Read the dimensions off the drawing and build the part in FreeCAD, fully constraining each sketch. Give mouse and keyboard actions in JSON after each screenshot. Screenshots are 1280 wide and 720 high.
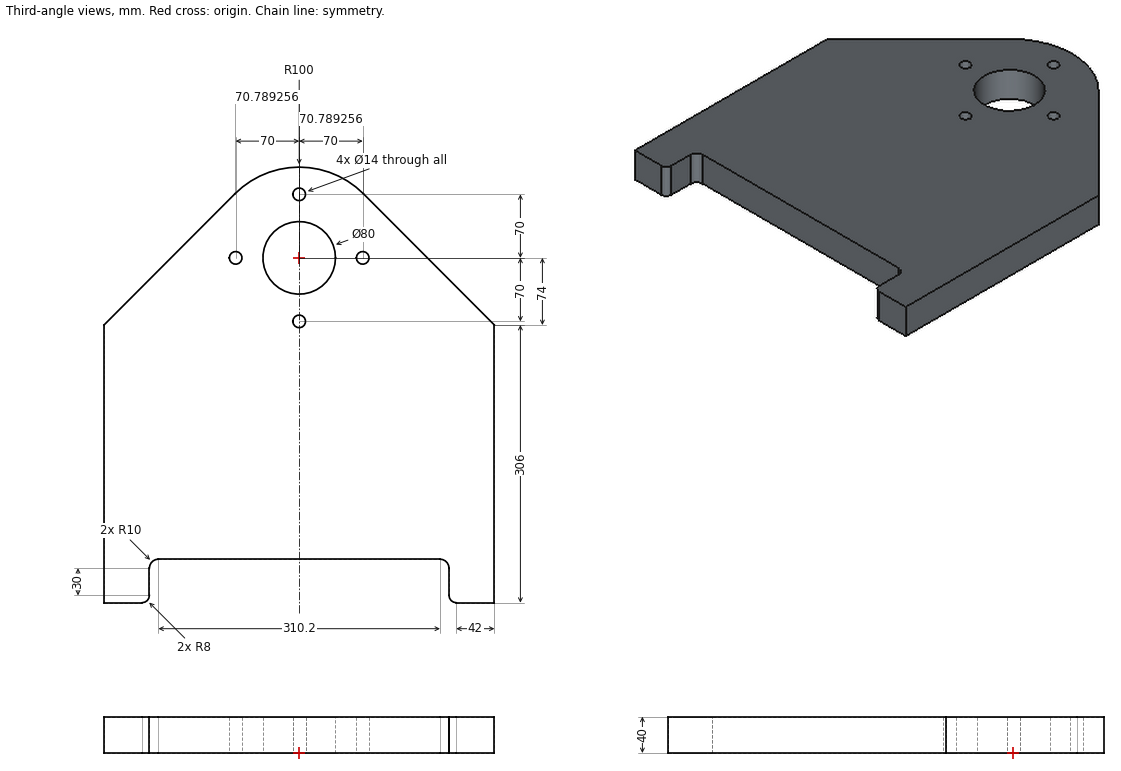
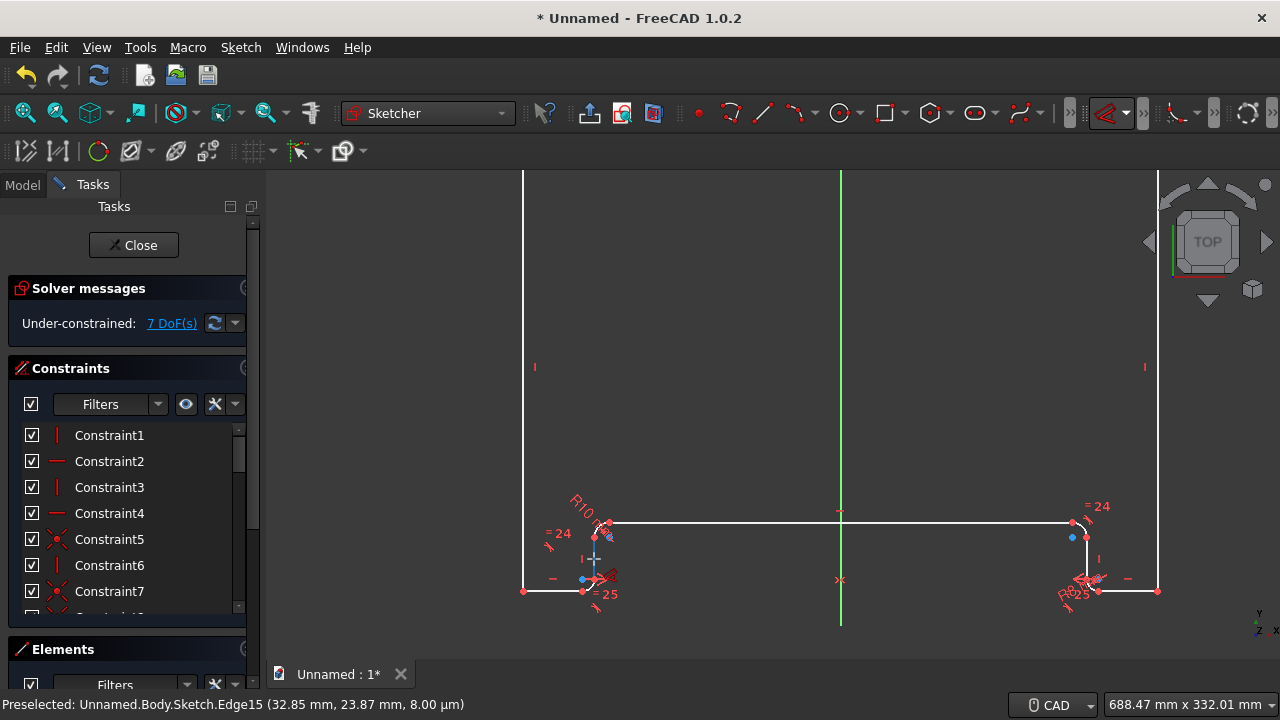
{"action": "left_click", "coordinate": [594, 558]}
{"action": "left_click", "coordinate": [560, 558]}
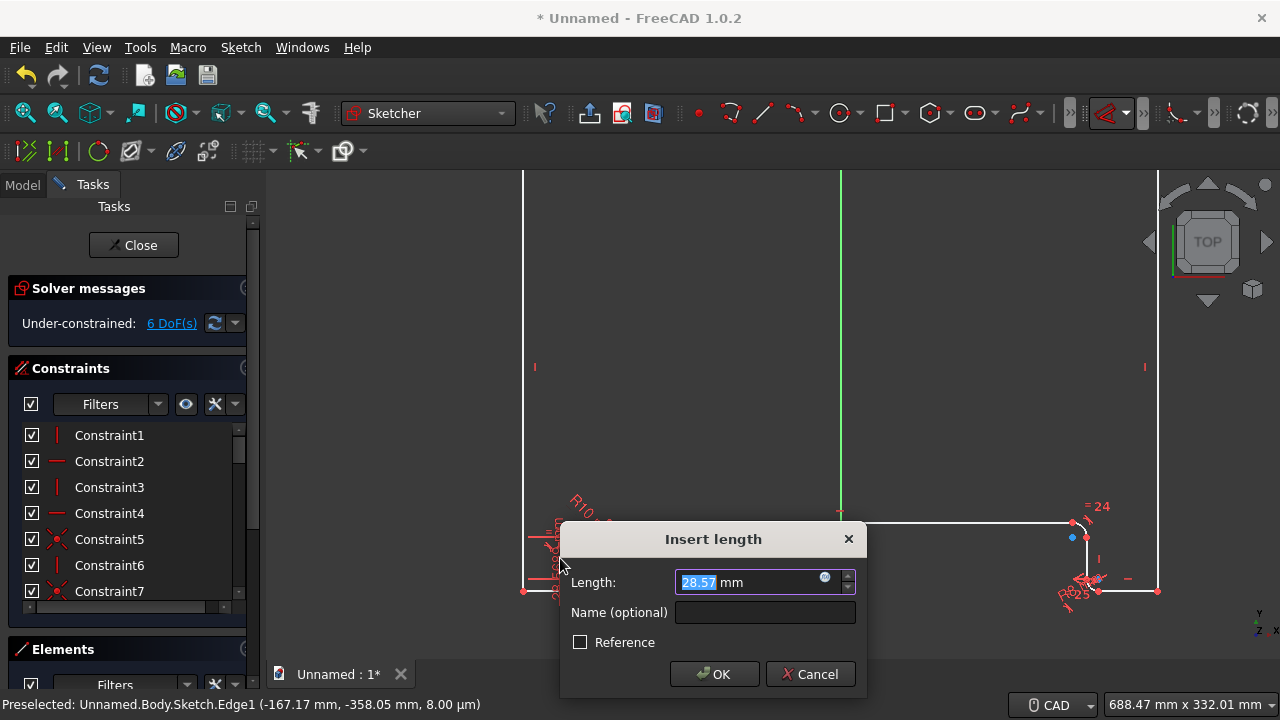
{"action": "type", "text": "30"}
{"action": "key", "text": "Return"}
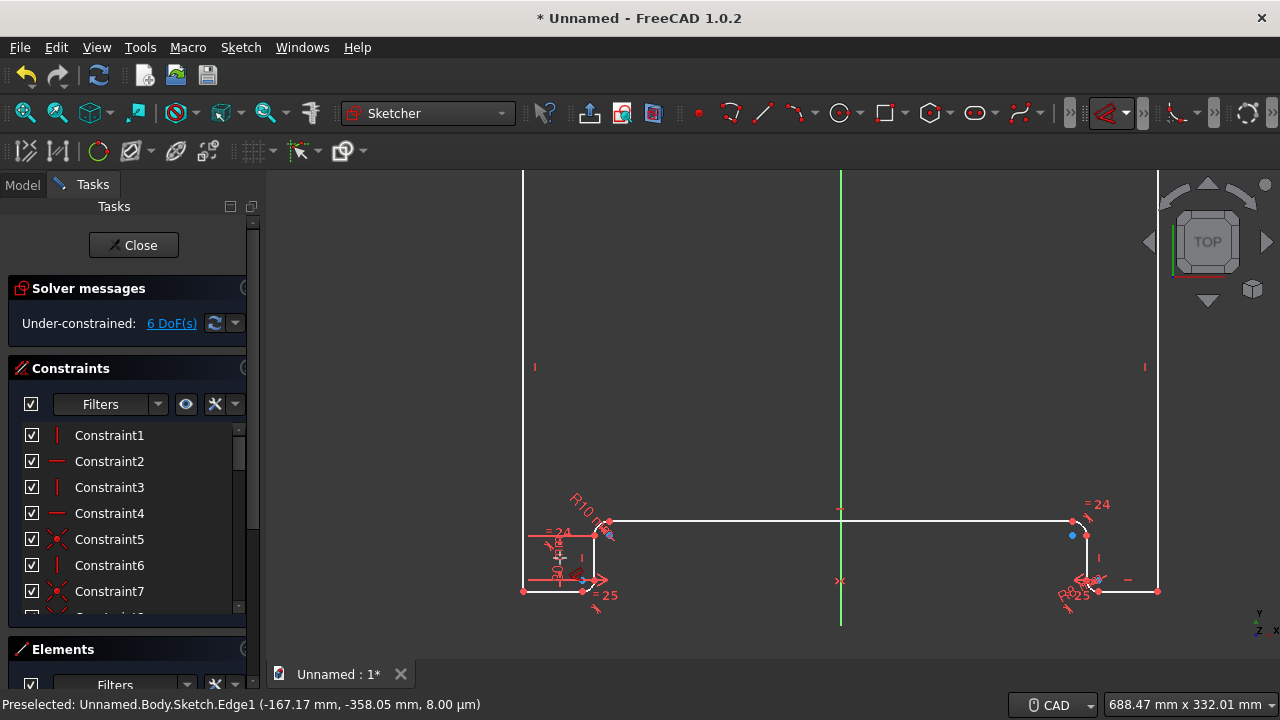
{"action": "left_click", "coordinate": [1110, 592]}
{"action": "left_click", "coordinate": [1107, 626]}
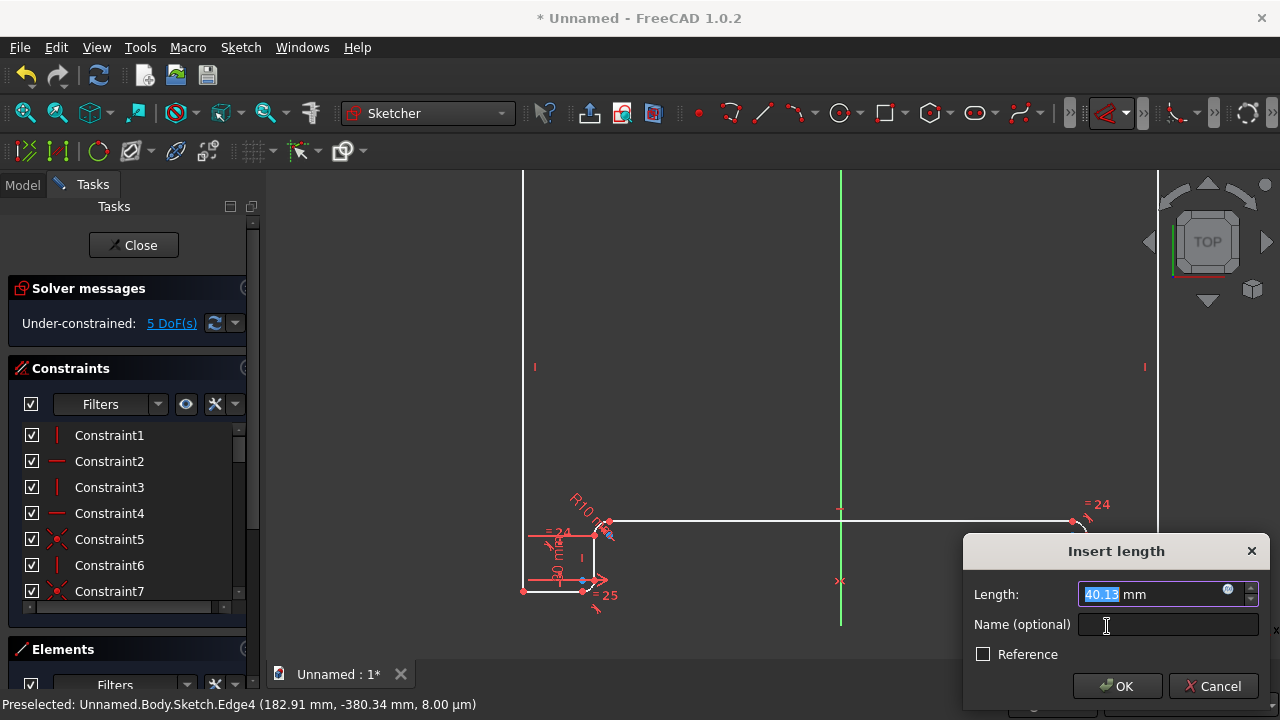
{"action": "type", "text": "42"}
{"action": "key", "text": "Return"}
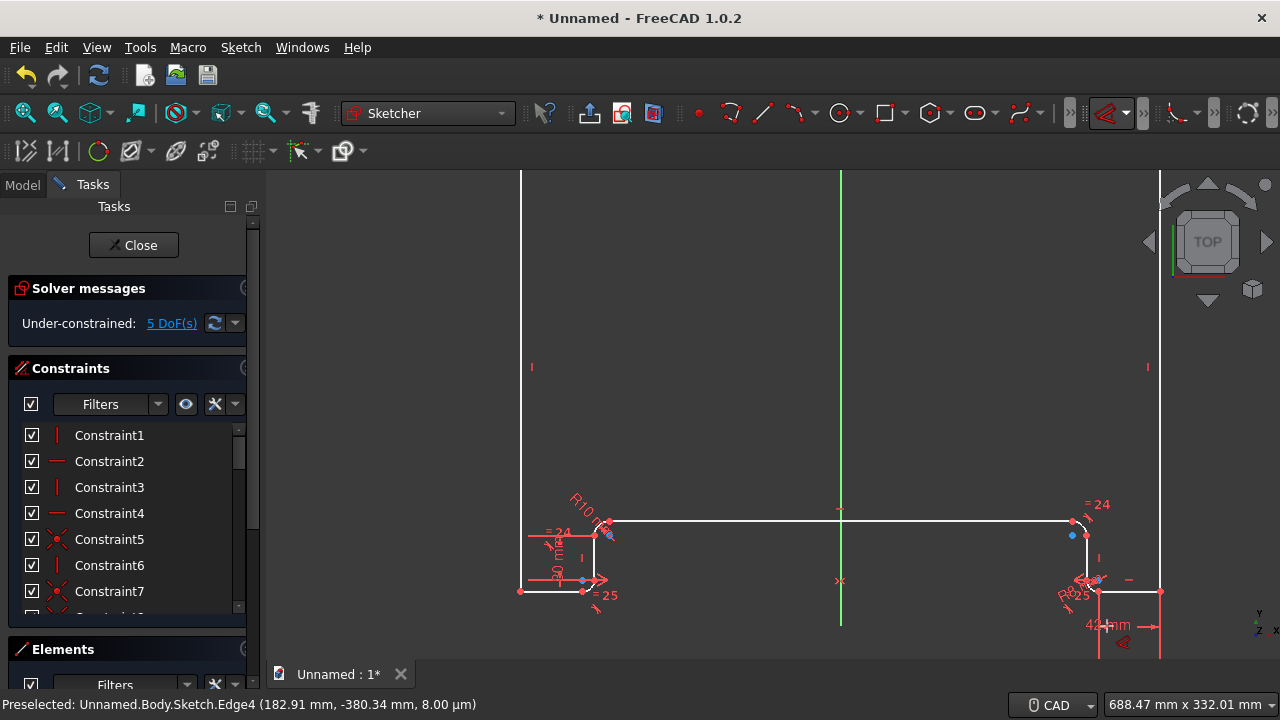
{"action": "scroll", "coordinate": [593, 559], "scroll_direction": "down", "scroll_amount": 4}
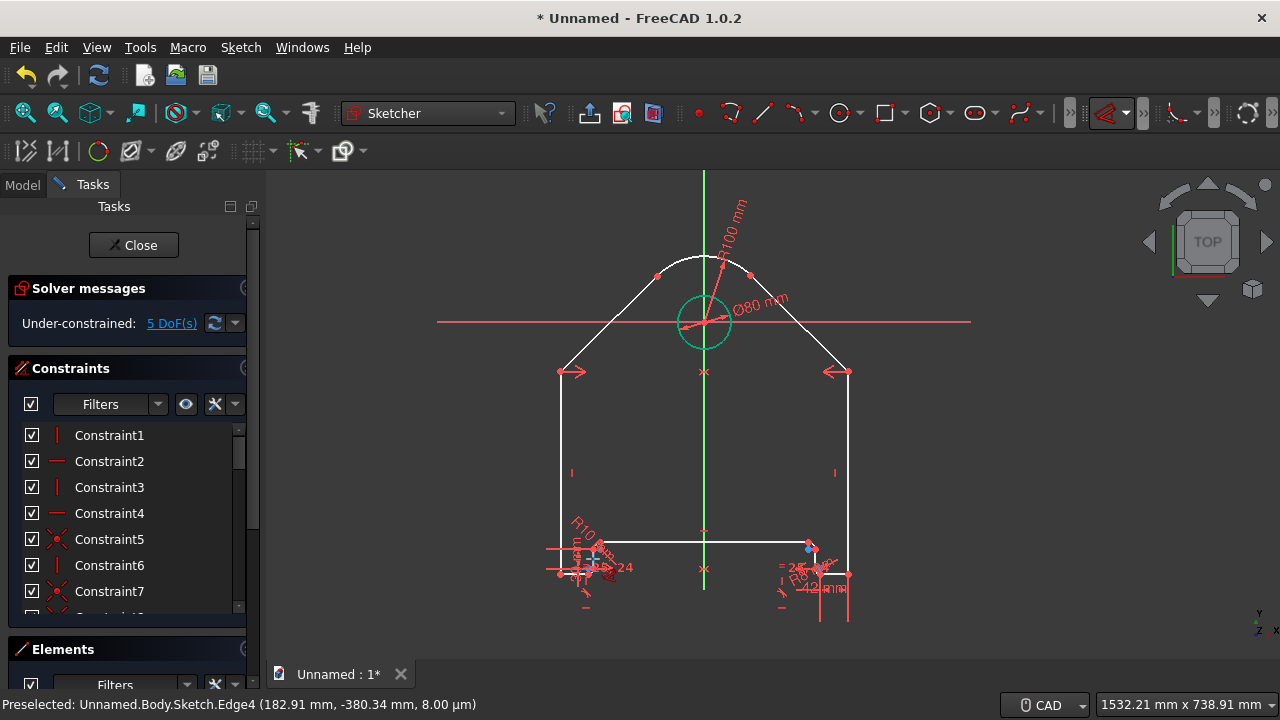
{"action": "left_click", "coordinate": [848, 513]}
{"action": "left_click", "coordinate": [882, 473]}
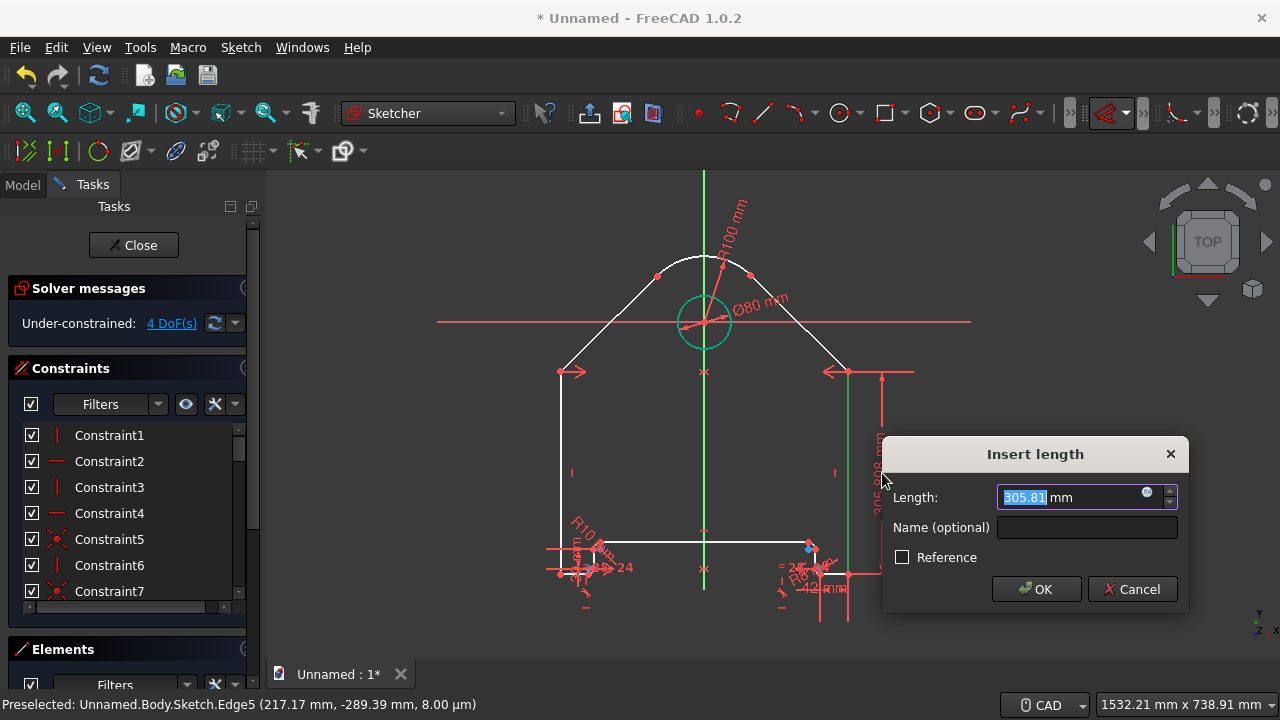
{"action": "type", "text": "306"}
{"action": "key", "text": "Return"}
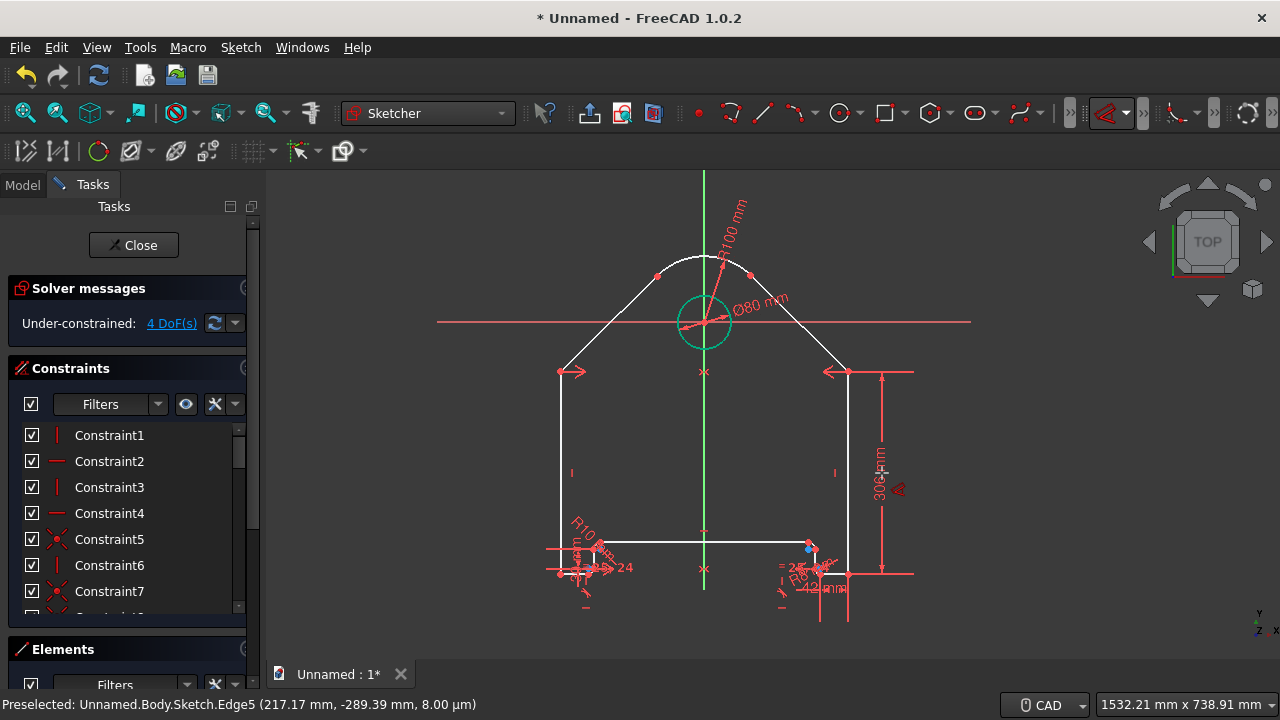
{"action": "left_click", "coordinate": [848, 372]}
{"action": "left_click", "coordinate": [882, 347]}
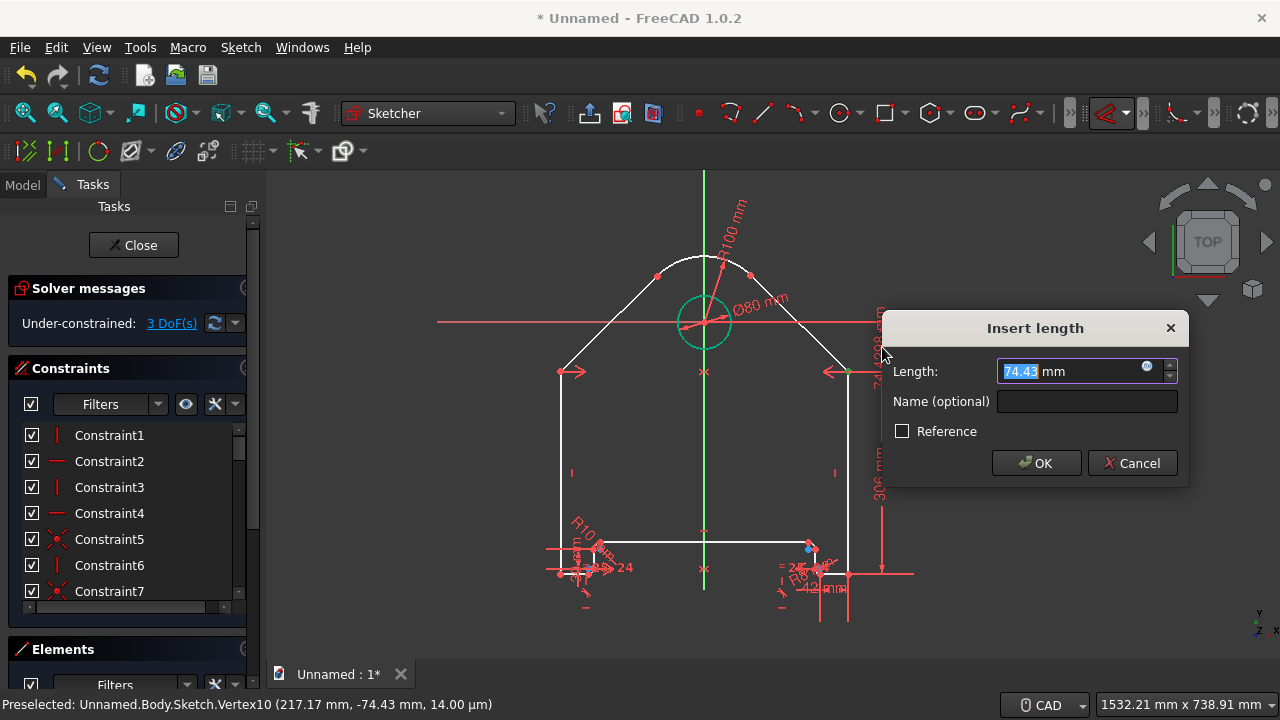
{"action": "type", "text": "74"}
{"action": "key", "text": "Return"}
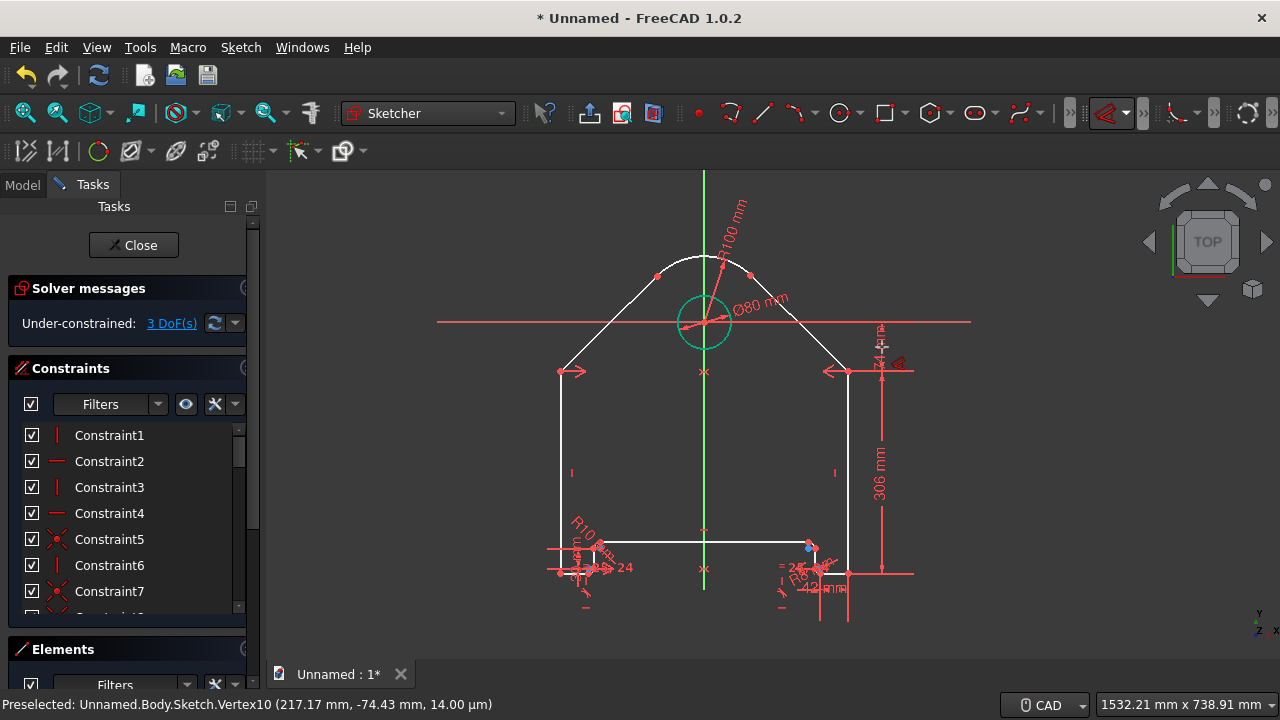
{"action": "left_click", "coordinate": [663, 542]}
{"action": "left_click", "coordinate": [657, 576]}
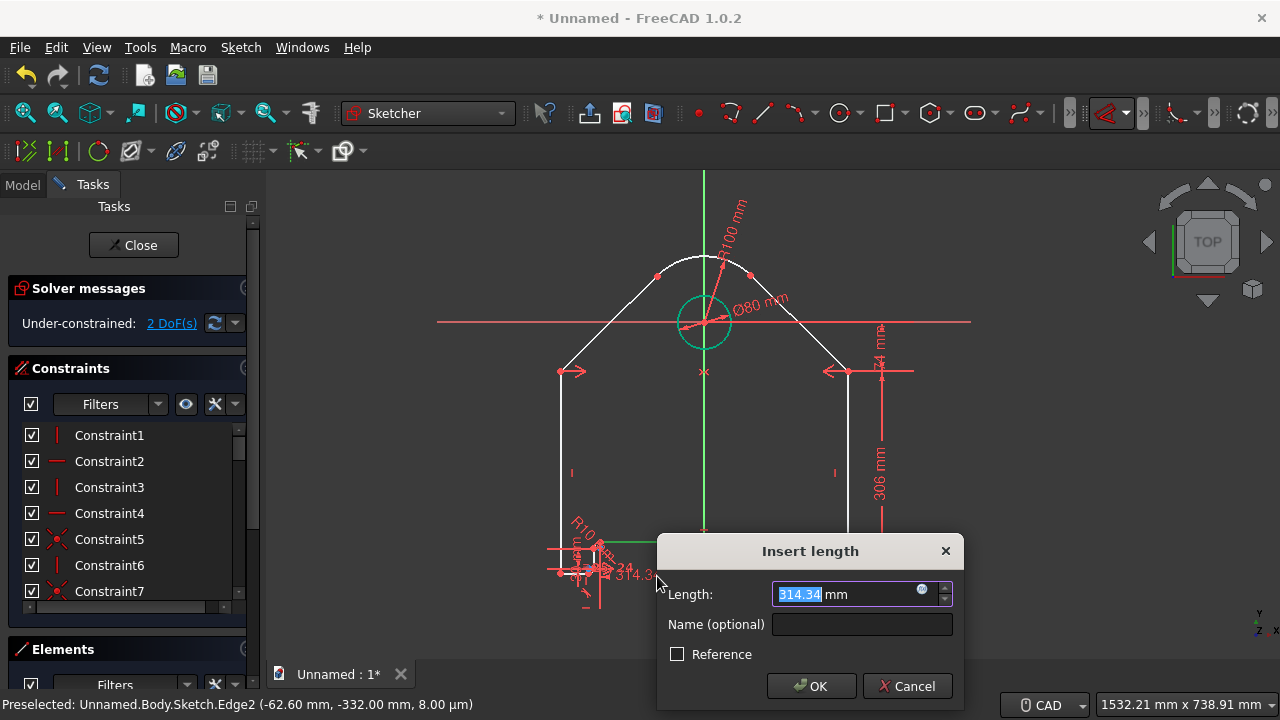
{"action": "type", "text": "310.2"}
{"action": "key", "text": "Return"}